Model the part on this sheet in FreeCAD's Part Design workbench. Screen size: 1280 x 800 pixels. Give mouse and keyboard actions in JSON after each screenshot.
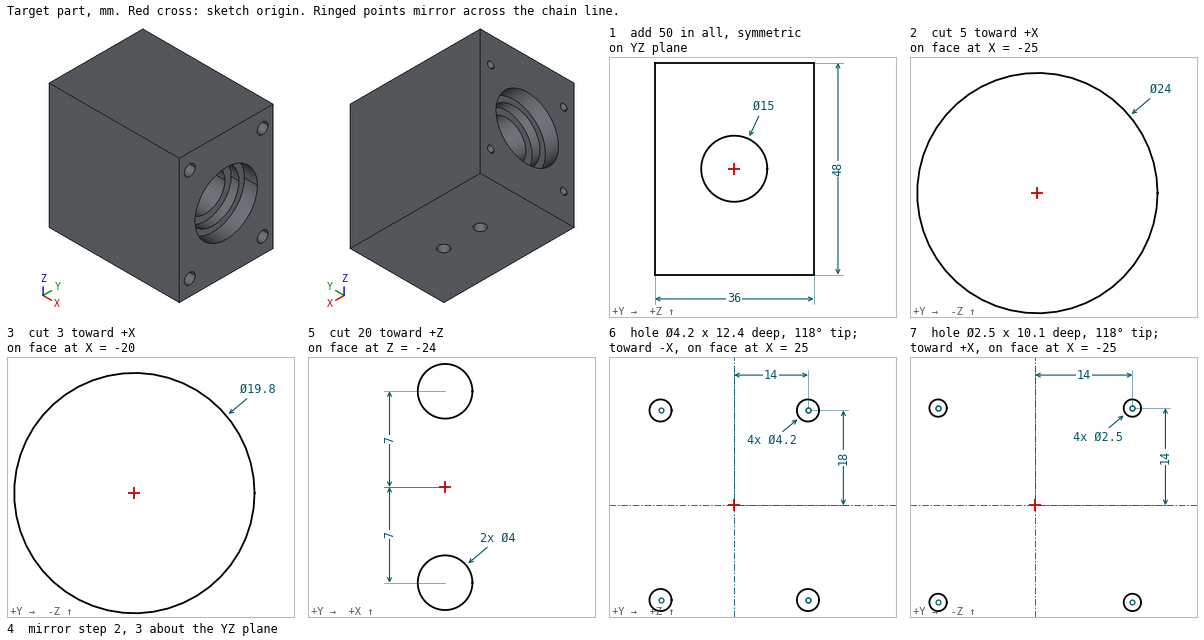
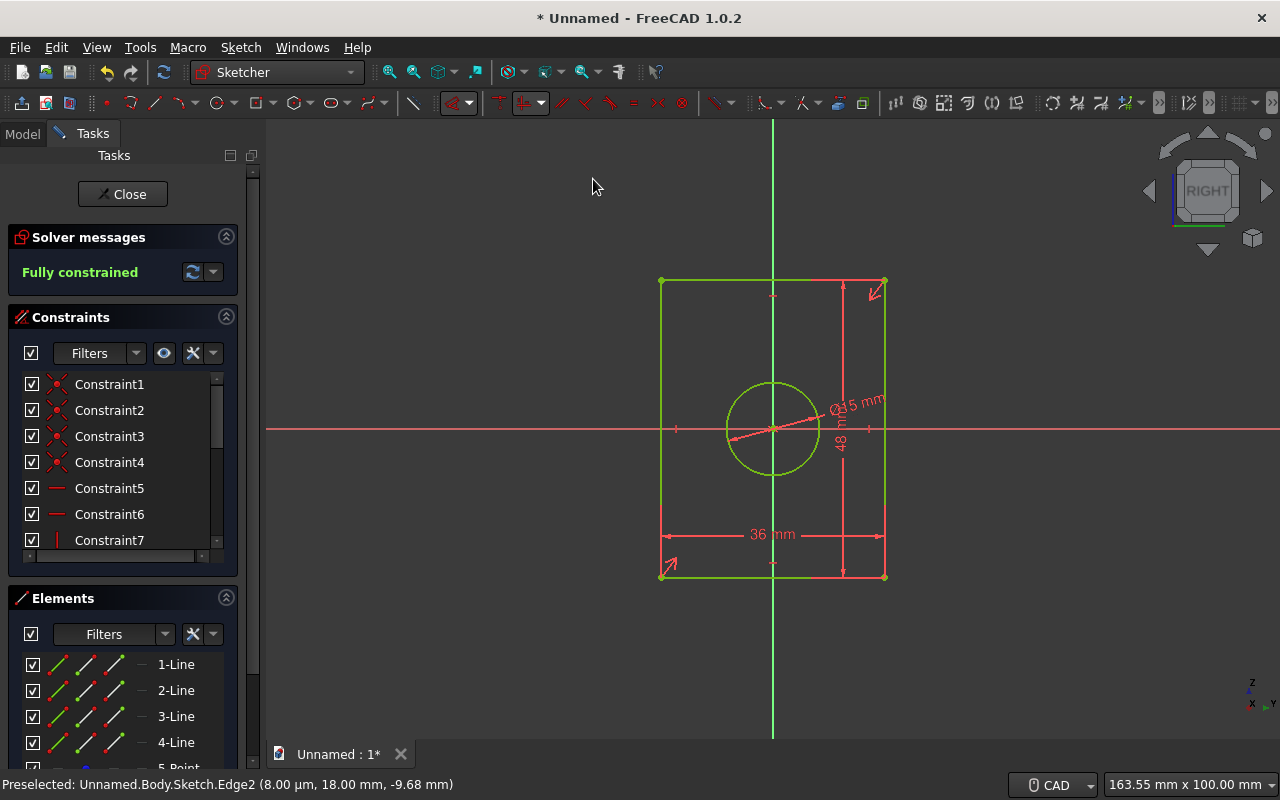
{"action": "left_click", "coordinate": [123, 194]}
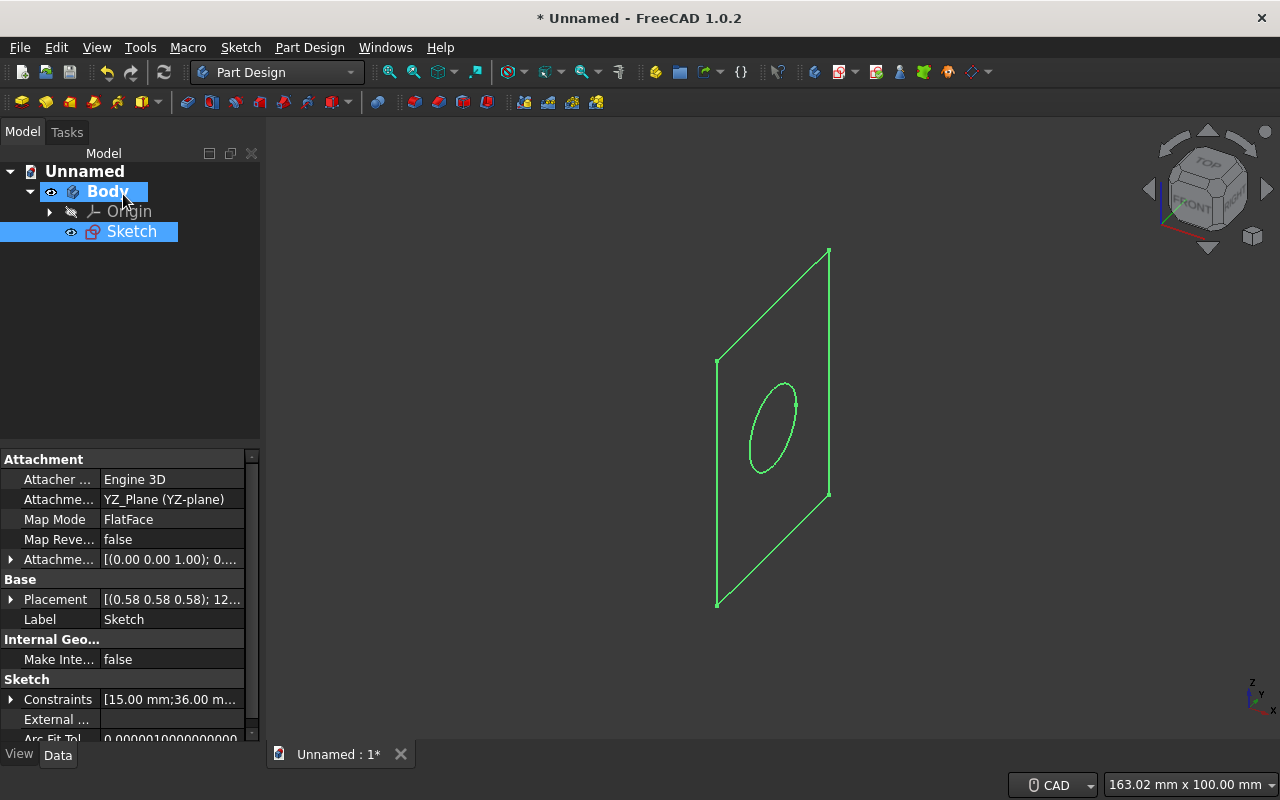
{"action": "left_click", "coordinate": [22, 102]}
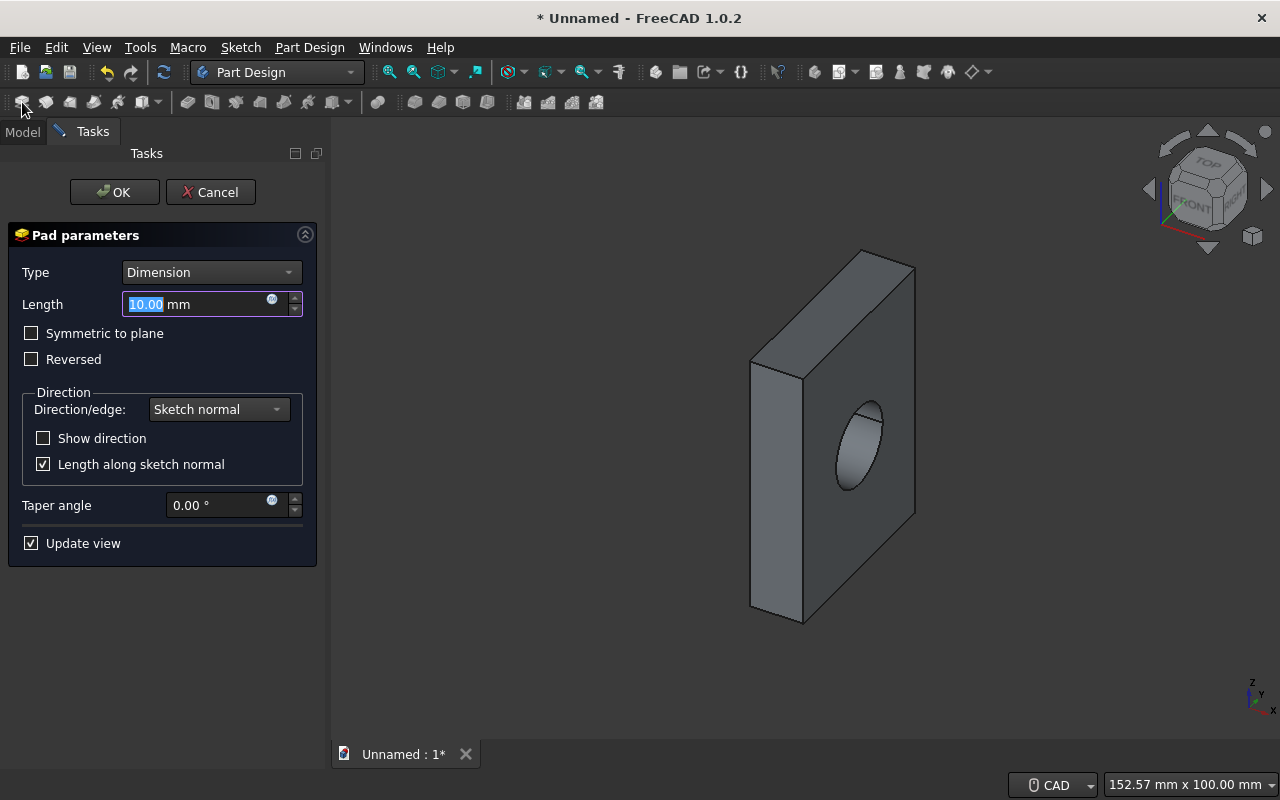
{"action": "type", "text": "50"}
{"action": "key", "text": "Tab"}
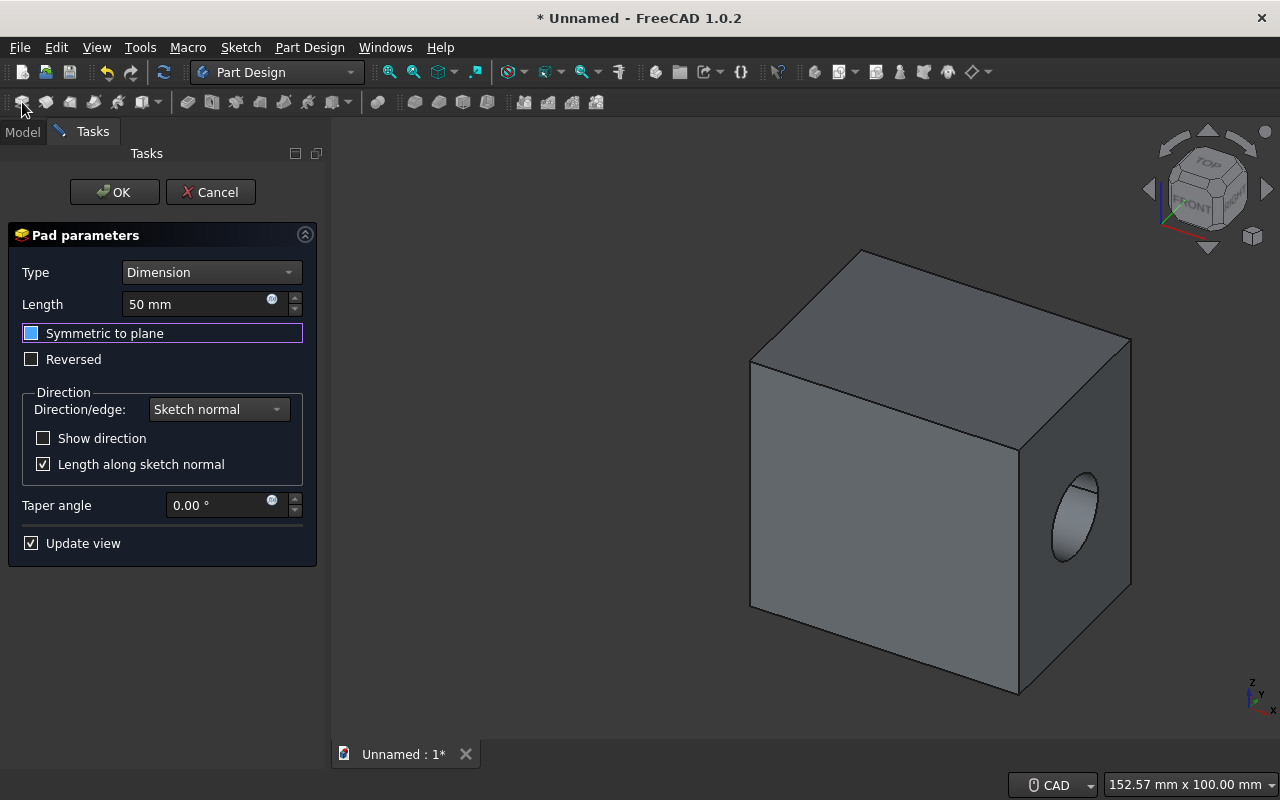
{"action": "left_click", "coordinate": [30, 333]}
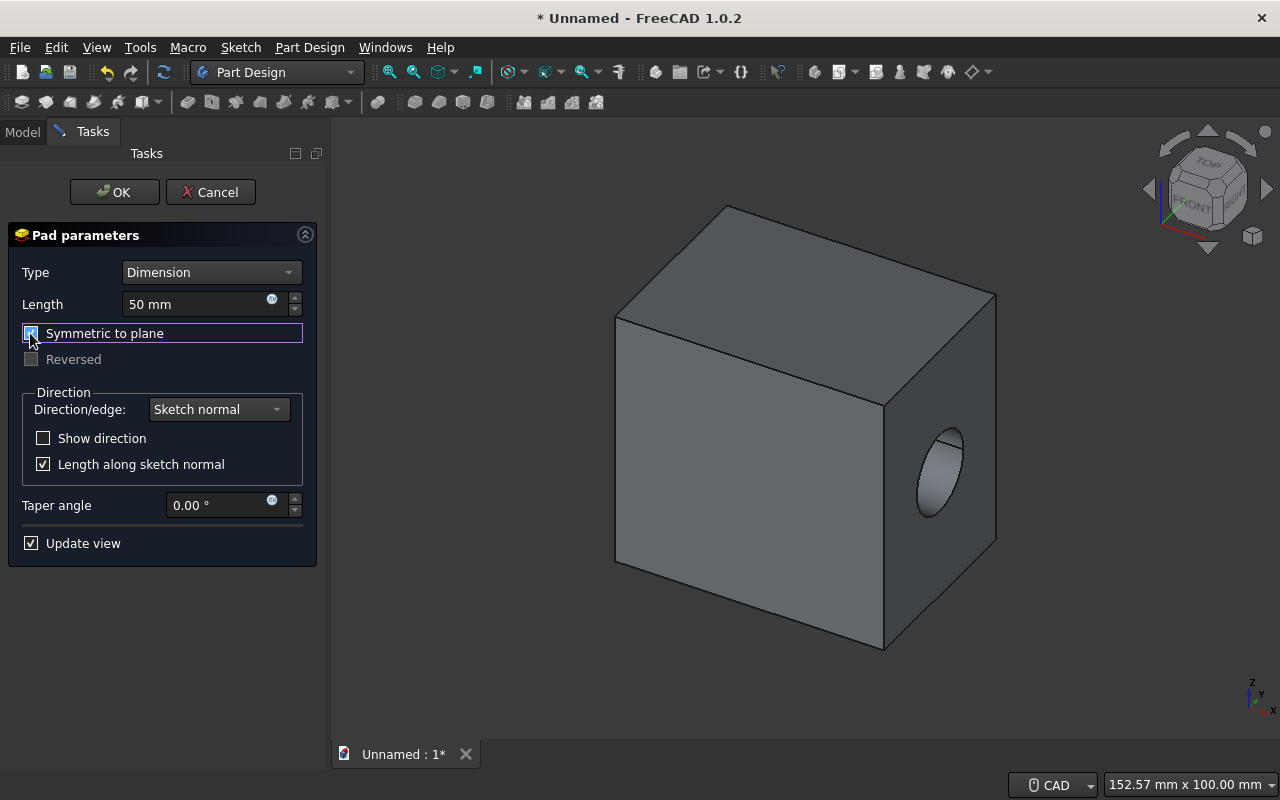
{"action": "left_click", "coordinate": [115, 192]}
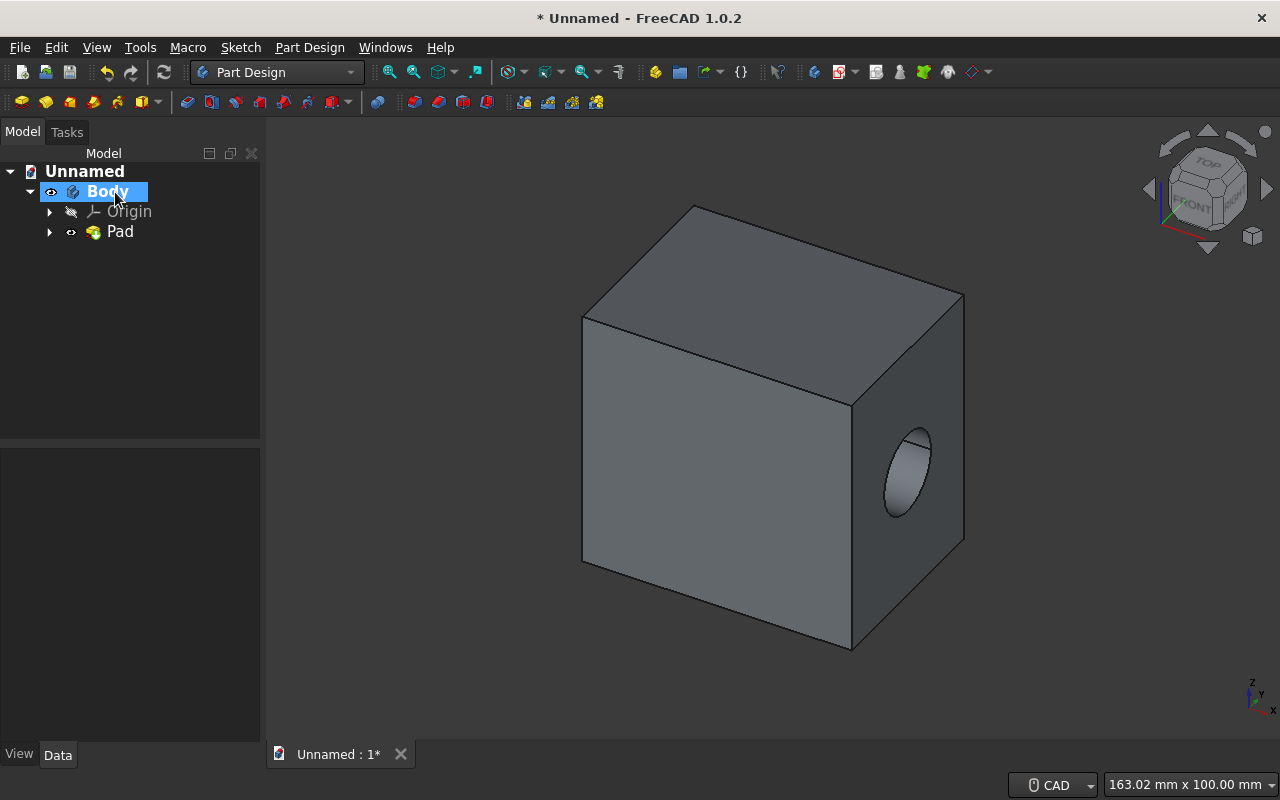
{"action": "key", "text": "6"}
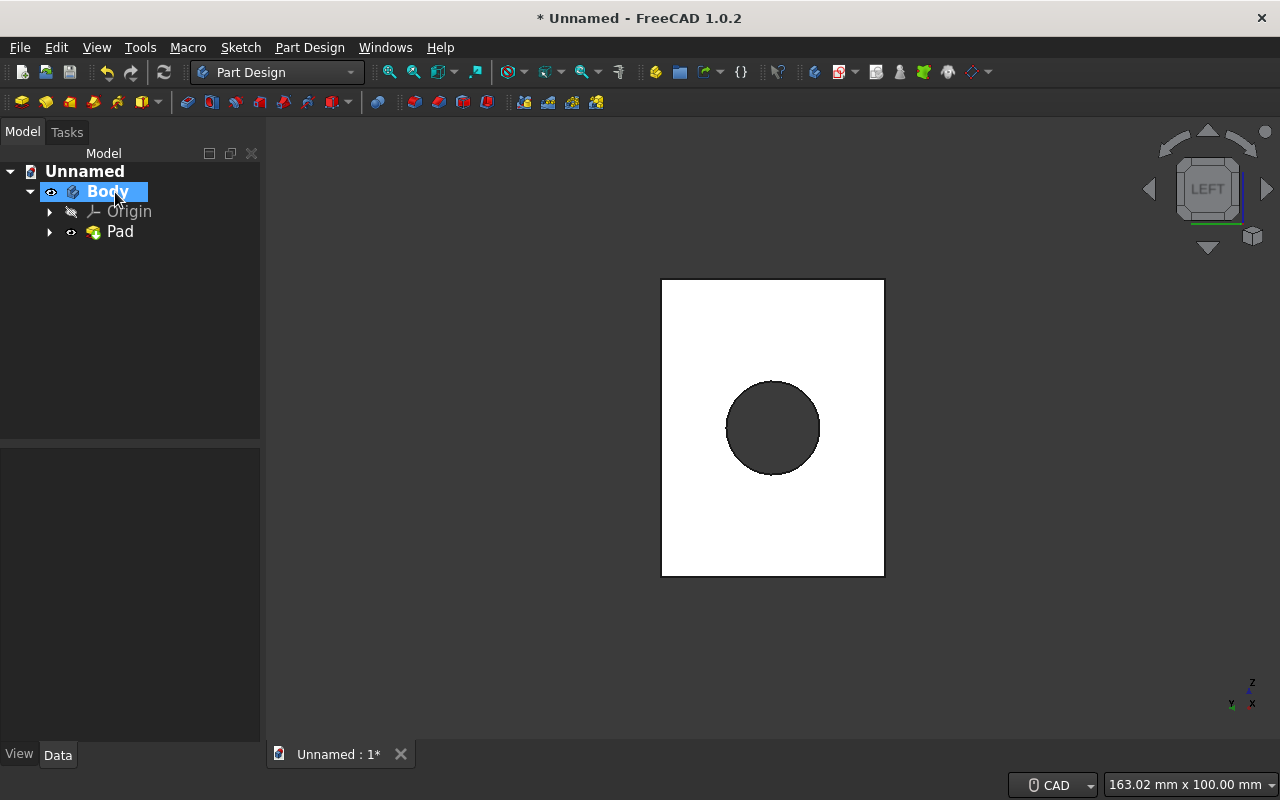
{"action": "left_click", "coordinate": [709, 512]}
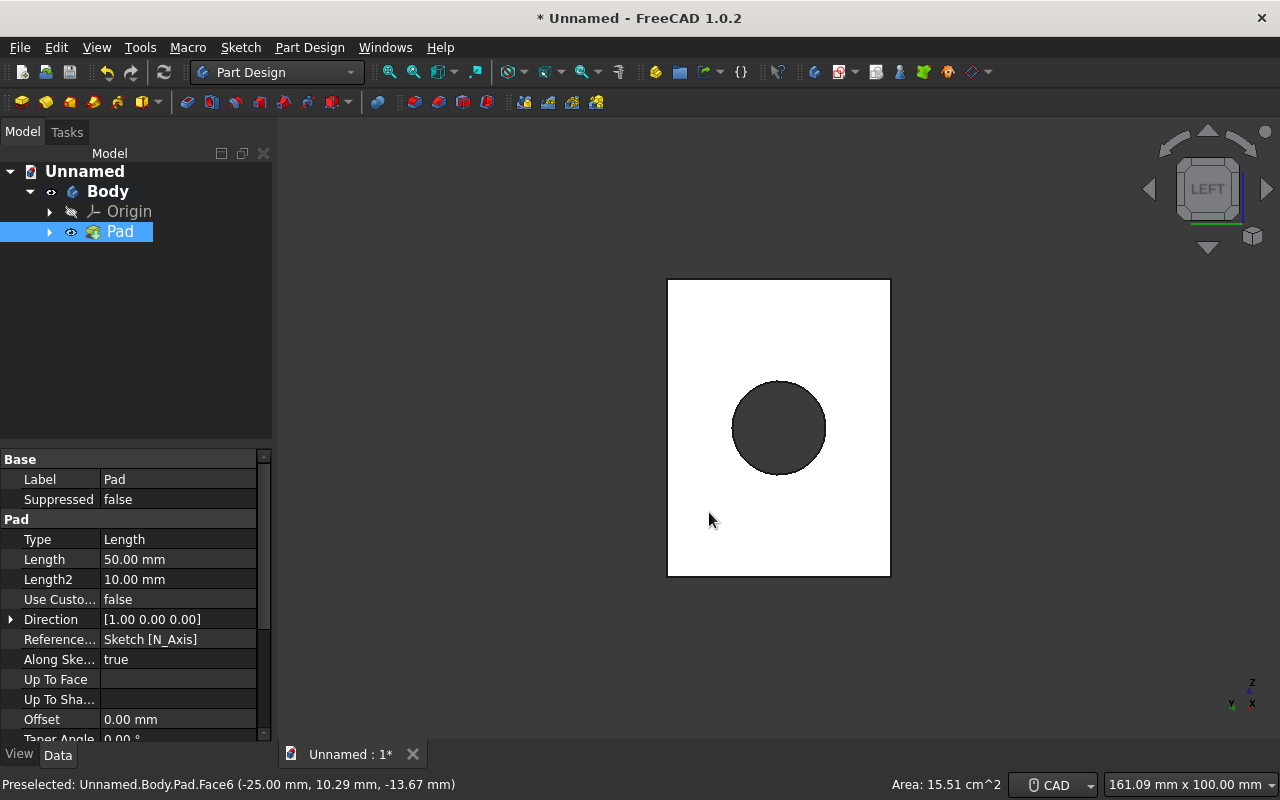
{"action": "left_click", "coordinate": [840, 72]}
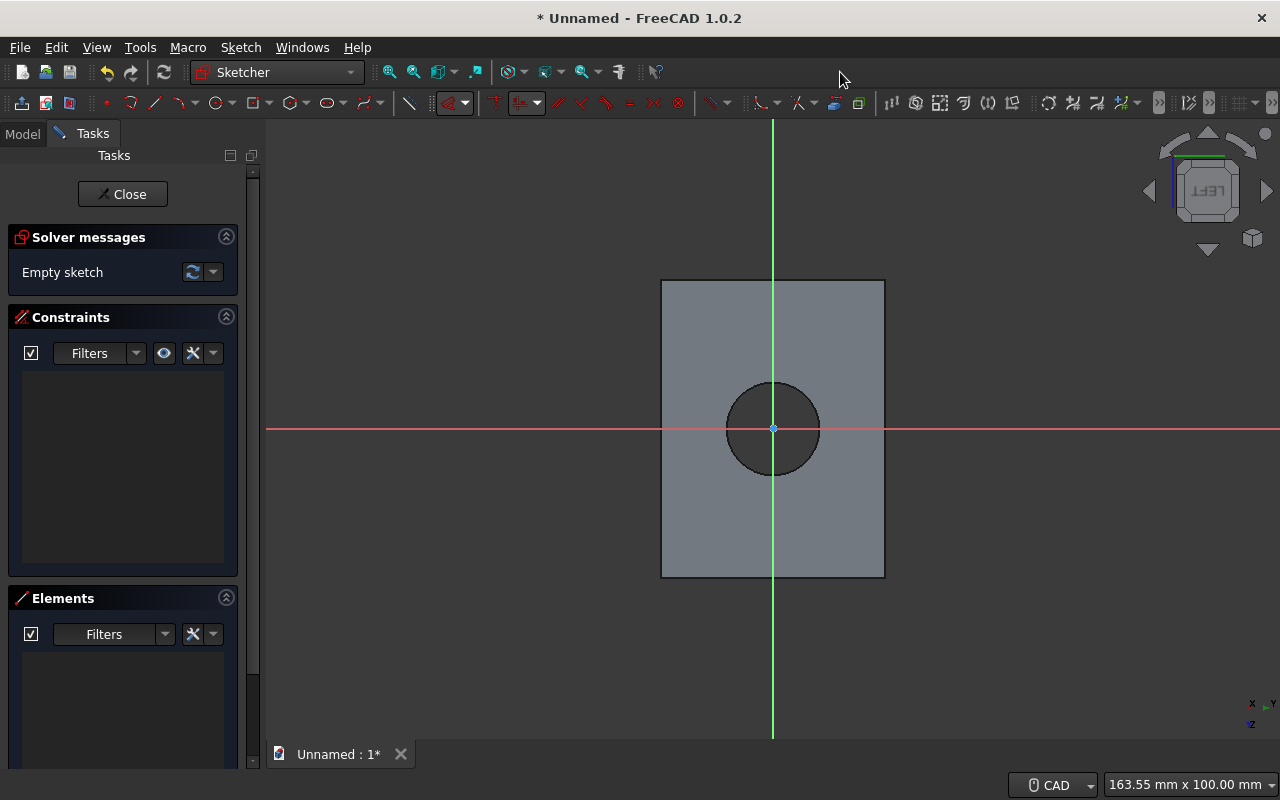
{"action": "scroll", "coordinate": [813, 429], "scroll_direction": "up", "scroll_amount": 5}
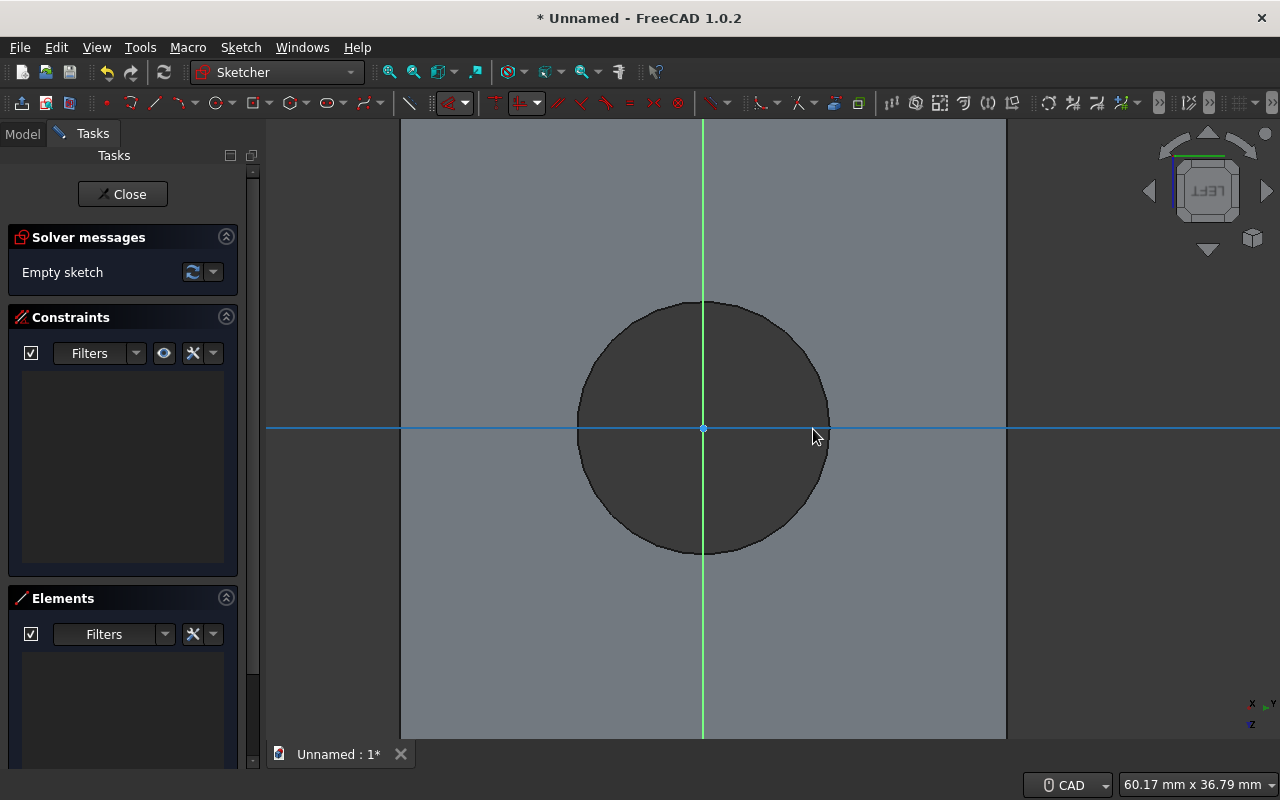
{"action": "left_click", "coordinate": [216, 104]}